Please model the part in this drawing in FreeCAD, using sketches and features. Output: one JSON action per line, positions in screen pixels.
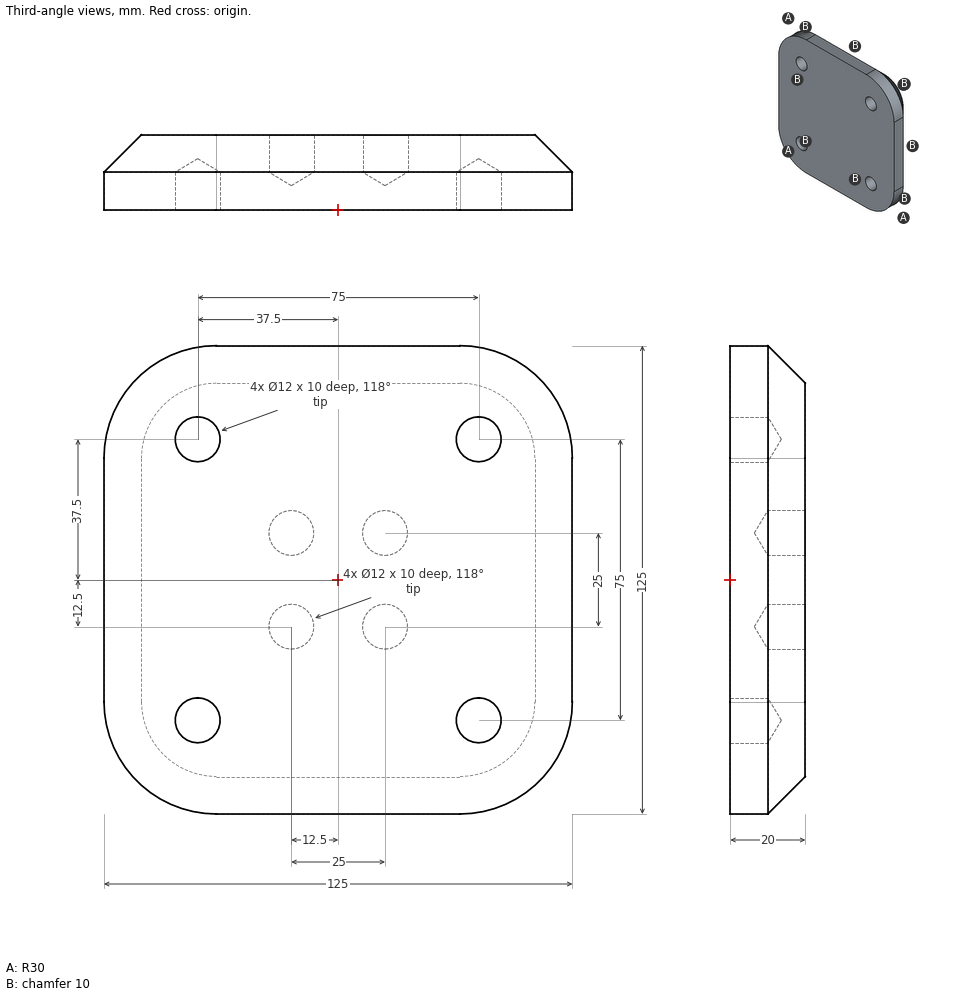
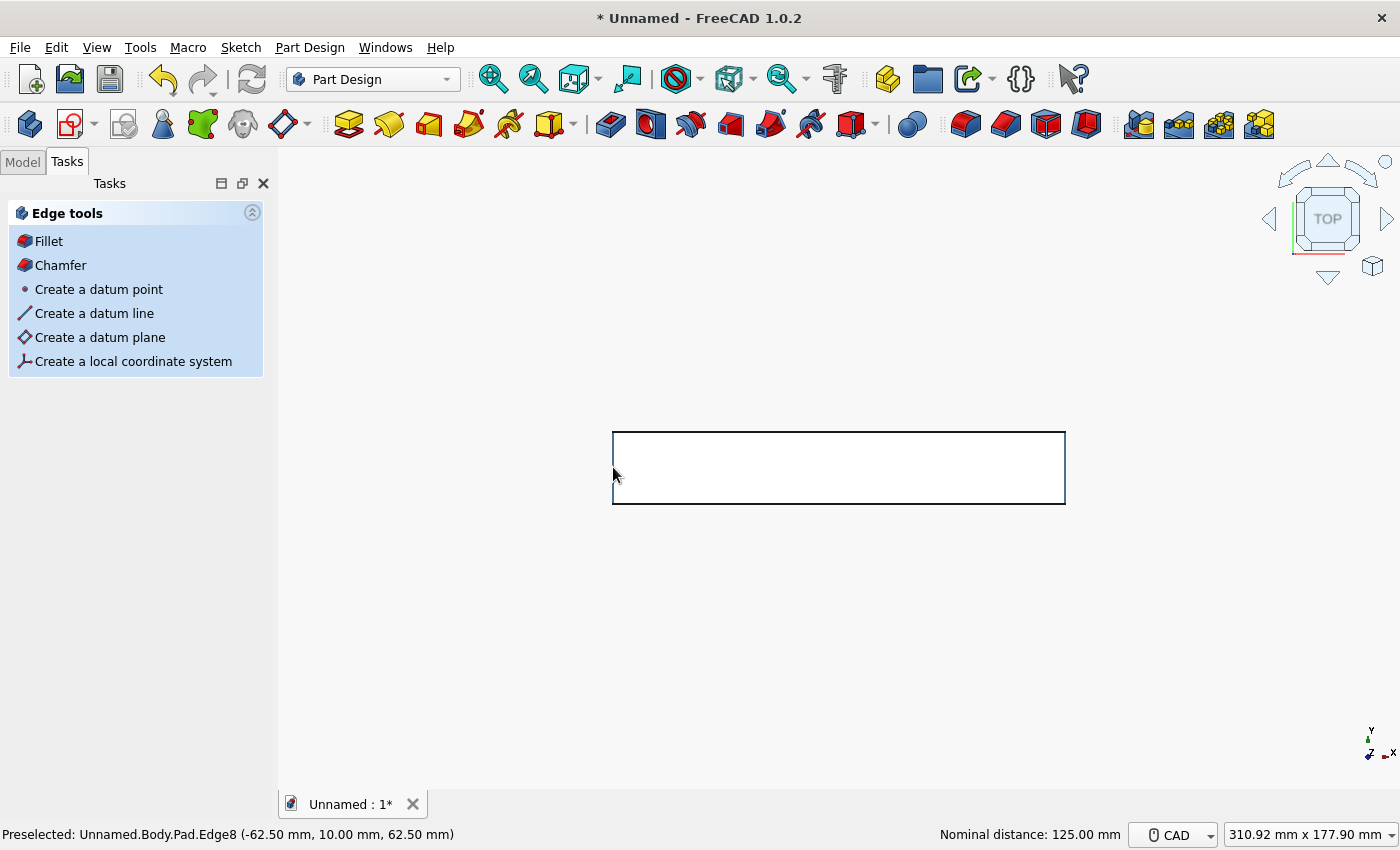
{"action": "key", "text": "1"}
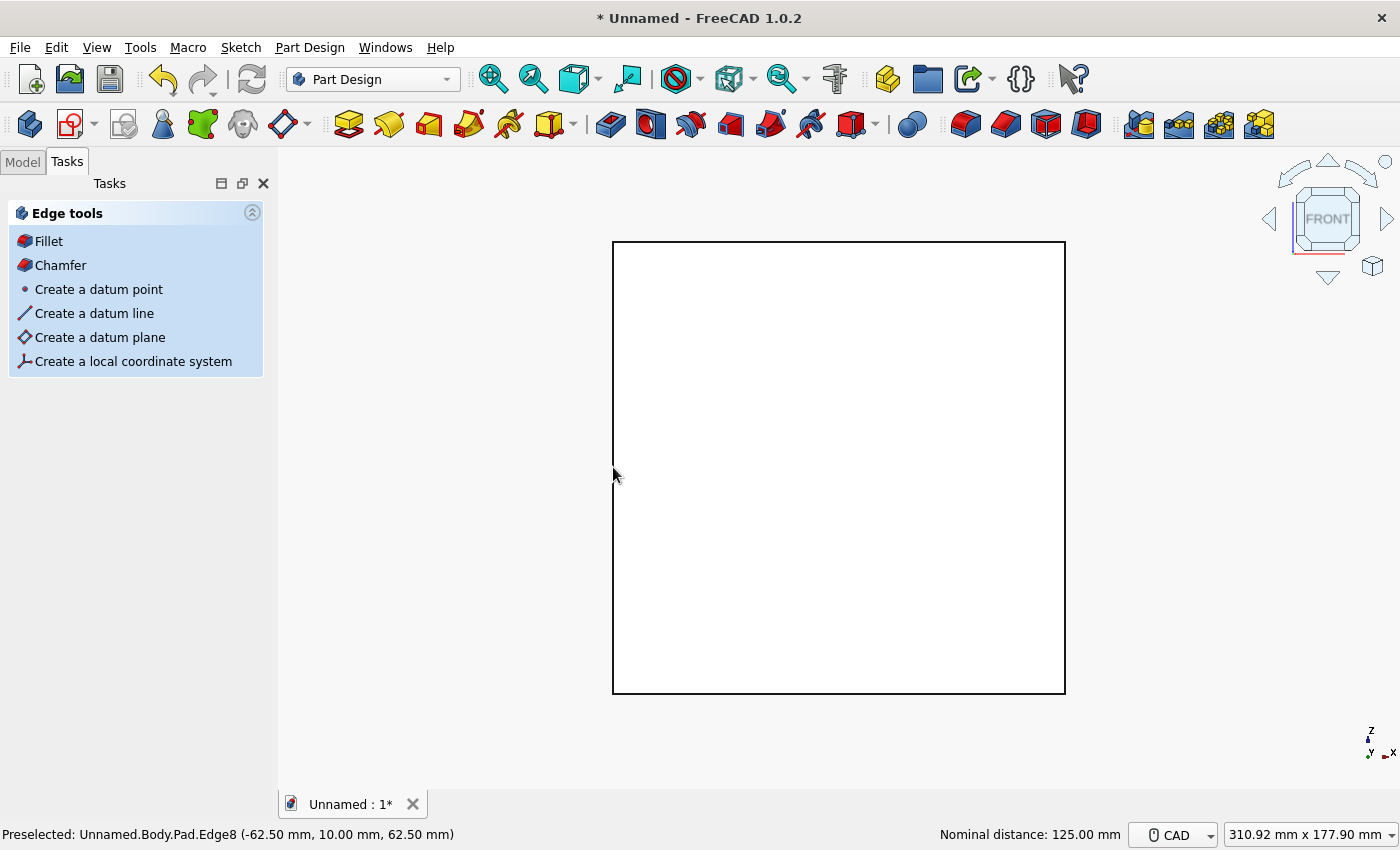
{"action": "key", "text": "3"}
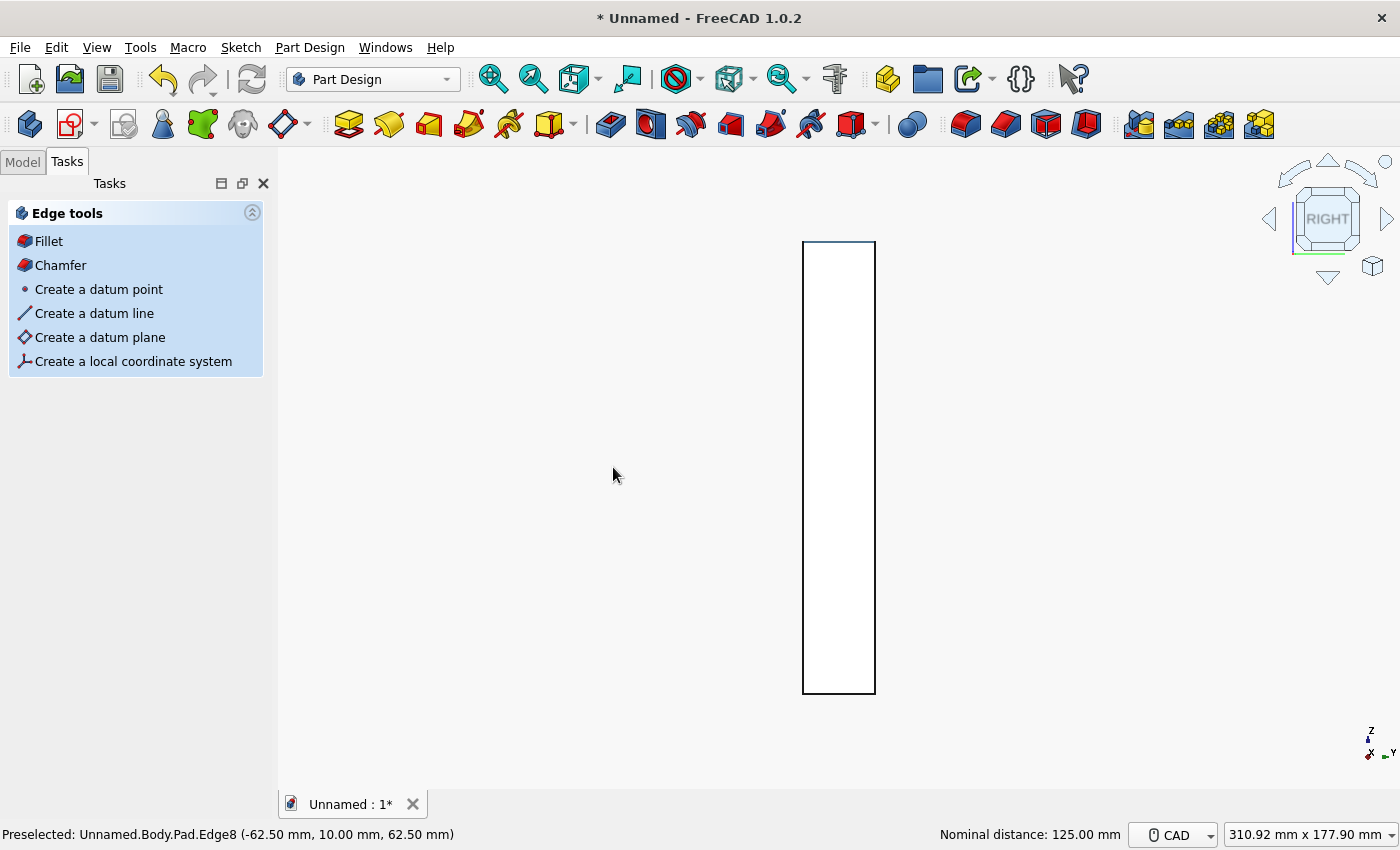
{"action": "left_click", "coordinate": [839, 693], "text": "ctrl"}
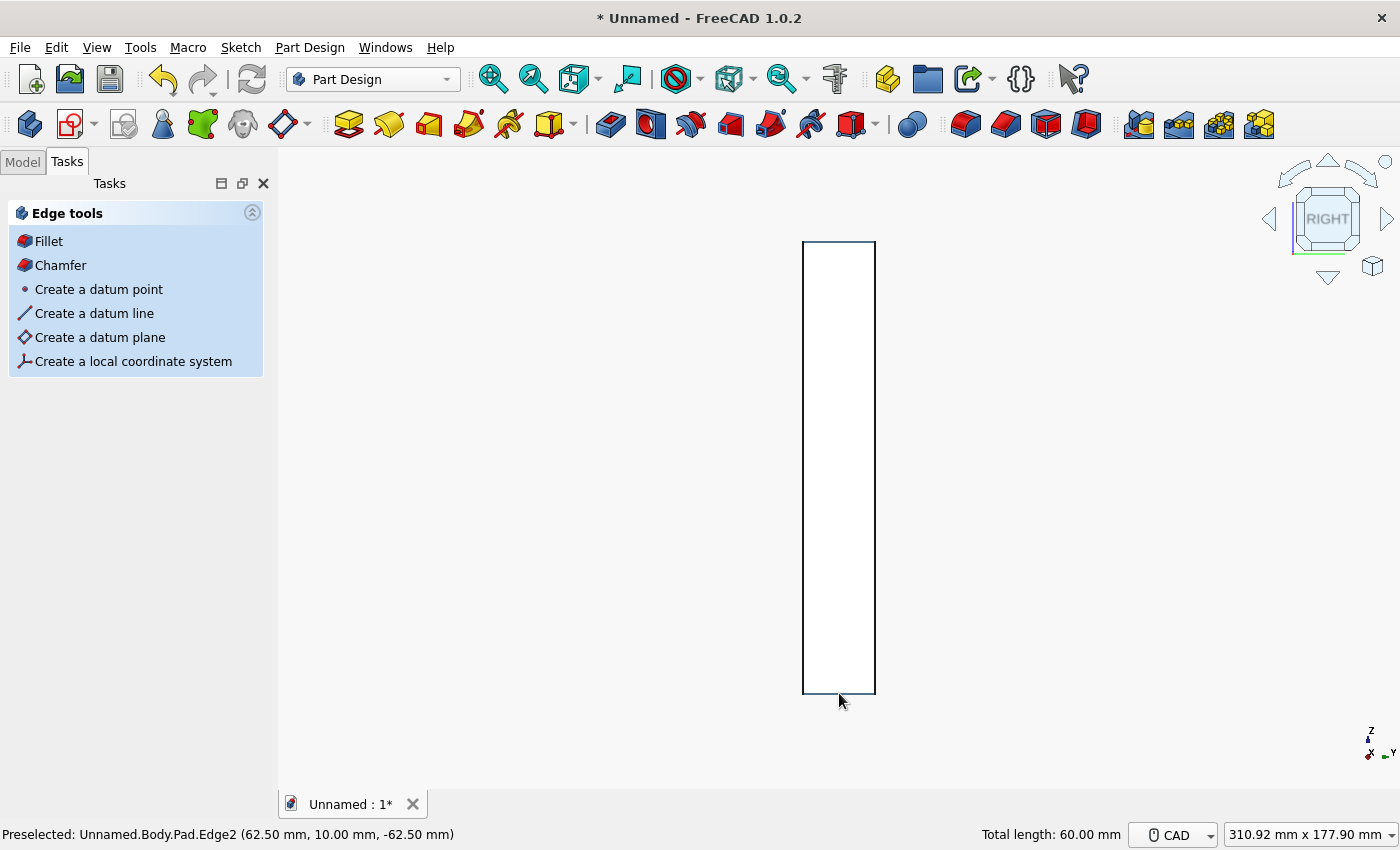
{"action": "key", "text": "5"}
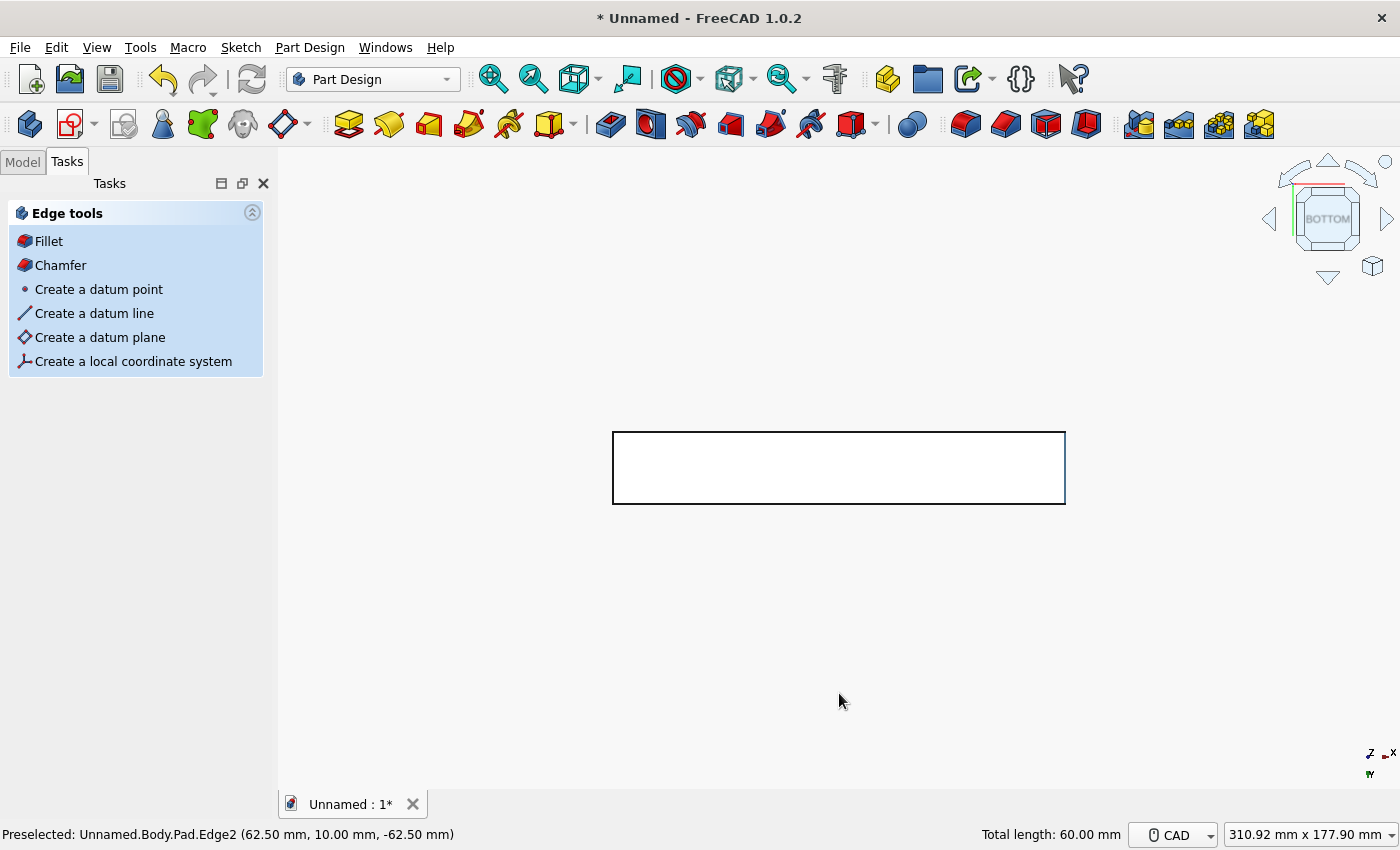
{"action": "key", "text": "v f"}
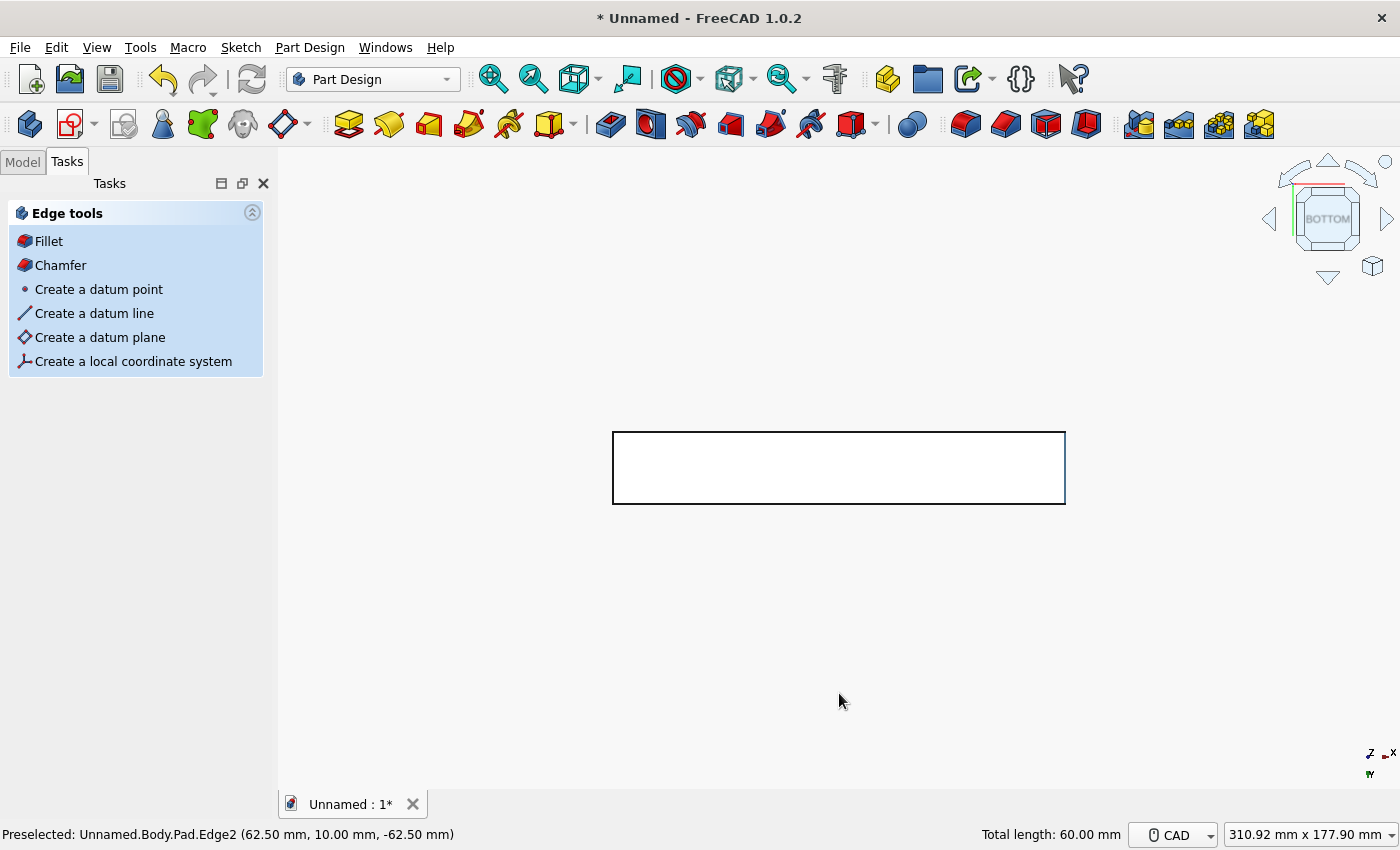
{"action": "left_click", "coordinate": [613, 467], "text": "ctrl"}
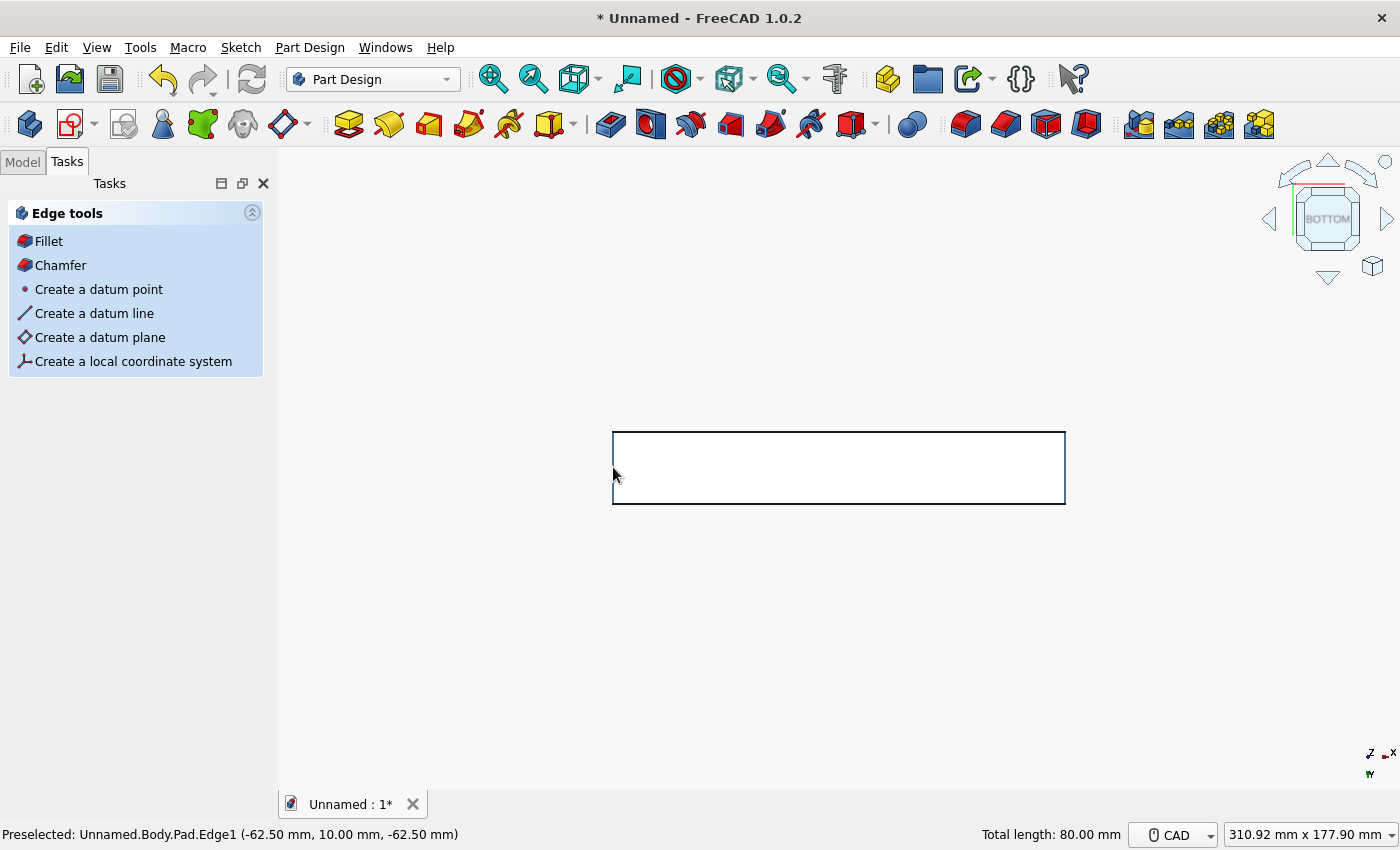
{"action": "left_click", "coordinate": [966, 124]}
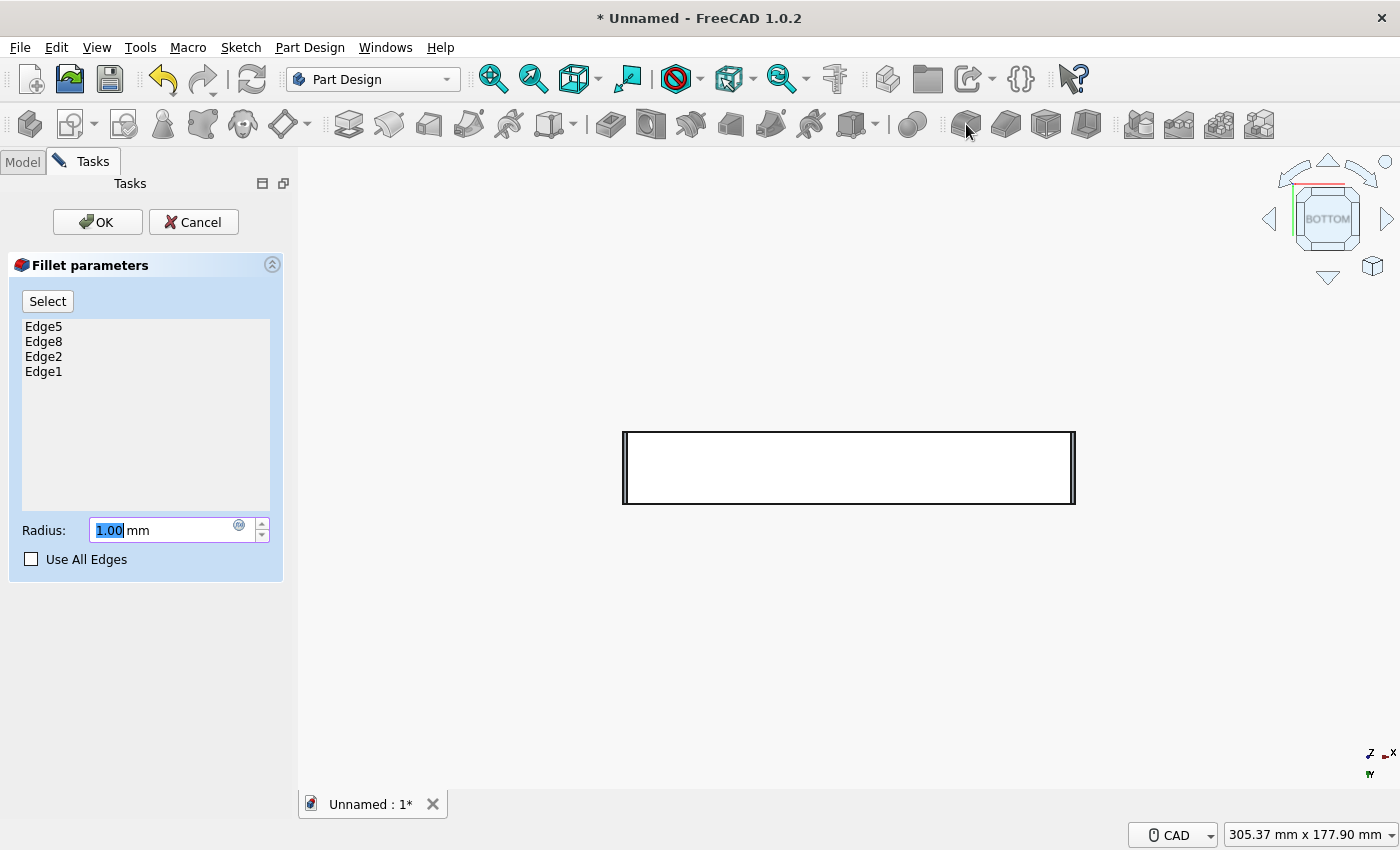
{"action": "type", "text": "30"}
{"action": "key", "text": "Tab"}